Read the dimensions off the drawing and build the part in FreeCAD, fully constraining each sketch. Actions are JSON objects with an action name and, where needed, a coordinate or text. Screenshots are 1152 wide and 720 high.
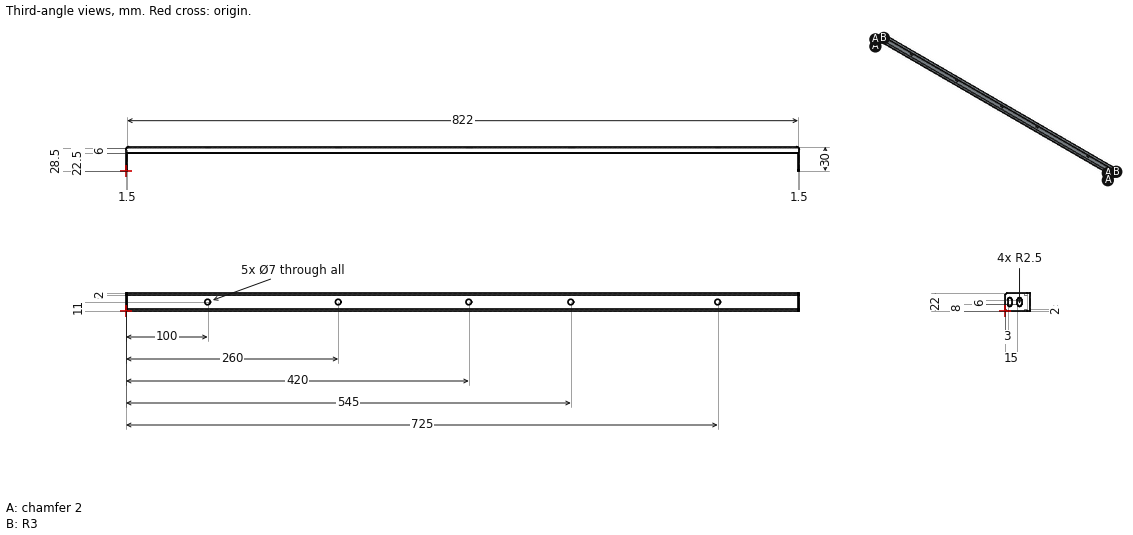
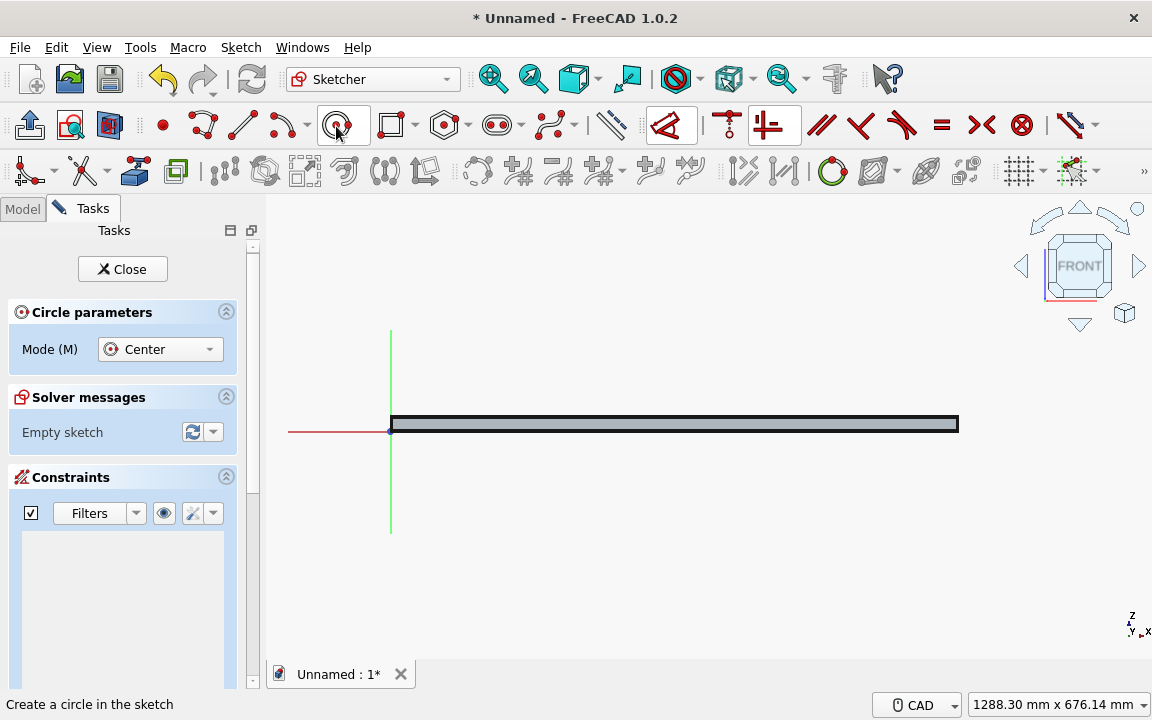
{"action": "scroll", "coordinate": [459, 424], "scroll_direction": "up", "scroll_amount": 12}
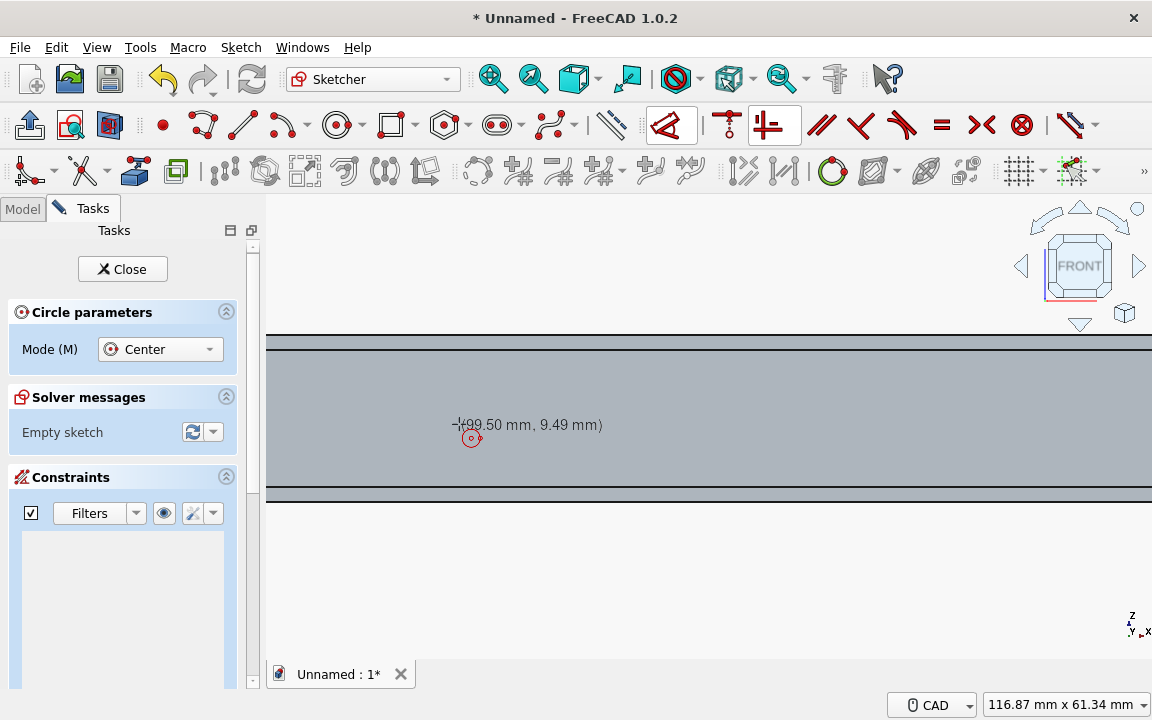
{"action": "scroll", "coordinate": [459, 424], "scroll_direction": "down", "scroll_amount": 12}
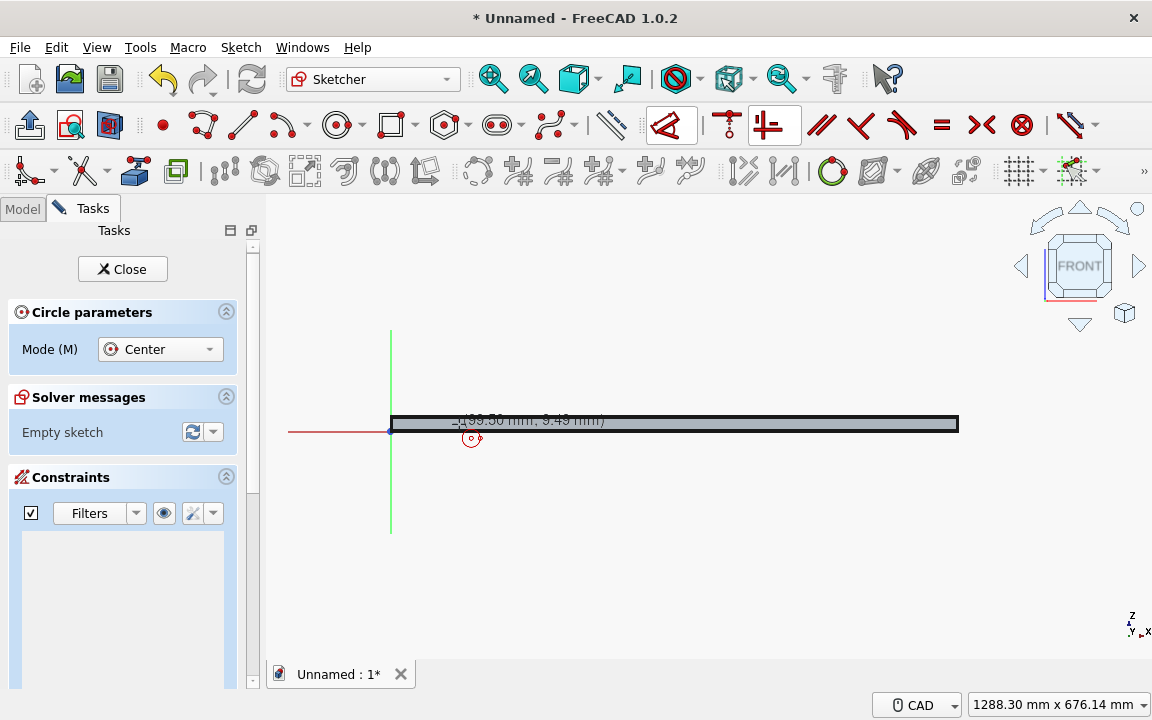
{"action": "scroll", "coordinate": [459, 424], "scroll_direction": "up", "scroll_amount": 4}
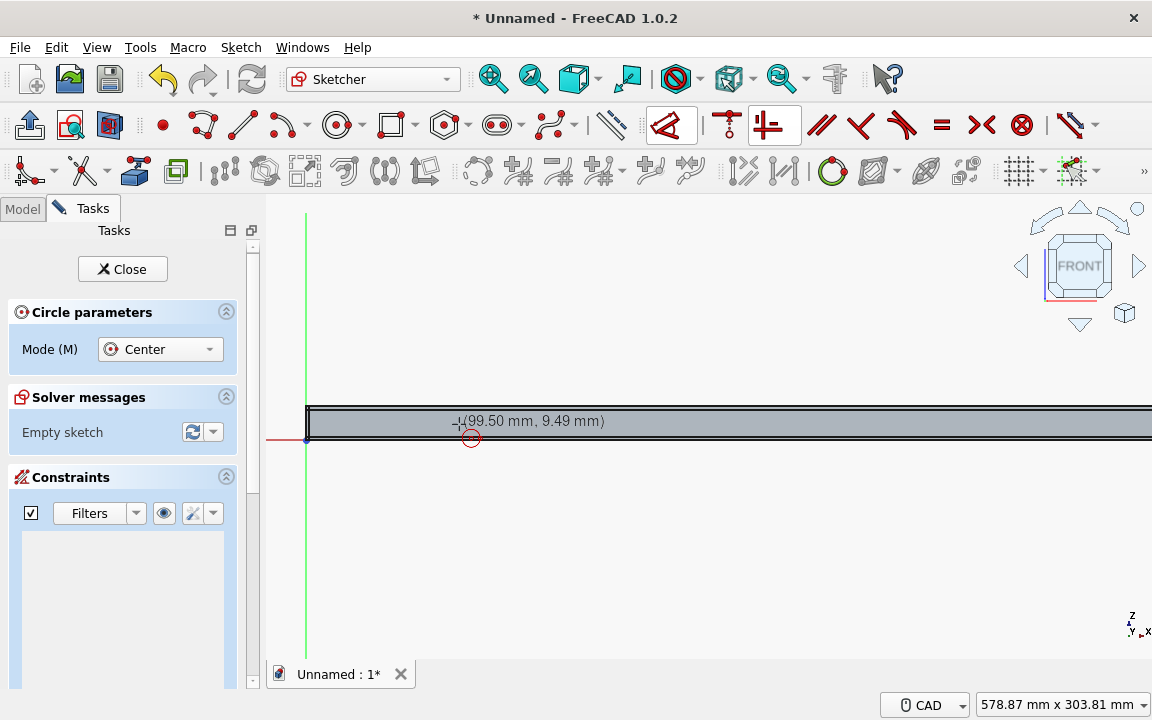
{"action": "left_click", "coordinate": [460, 423]}
{"action": "mouse_move", "coordinate": [463, 420]}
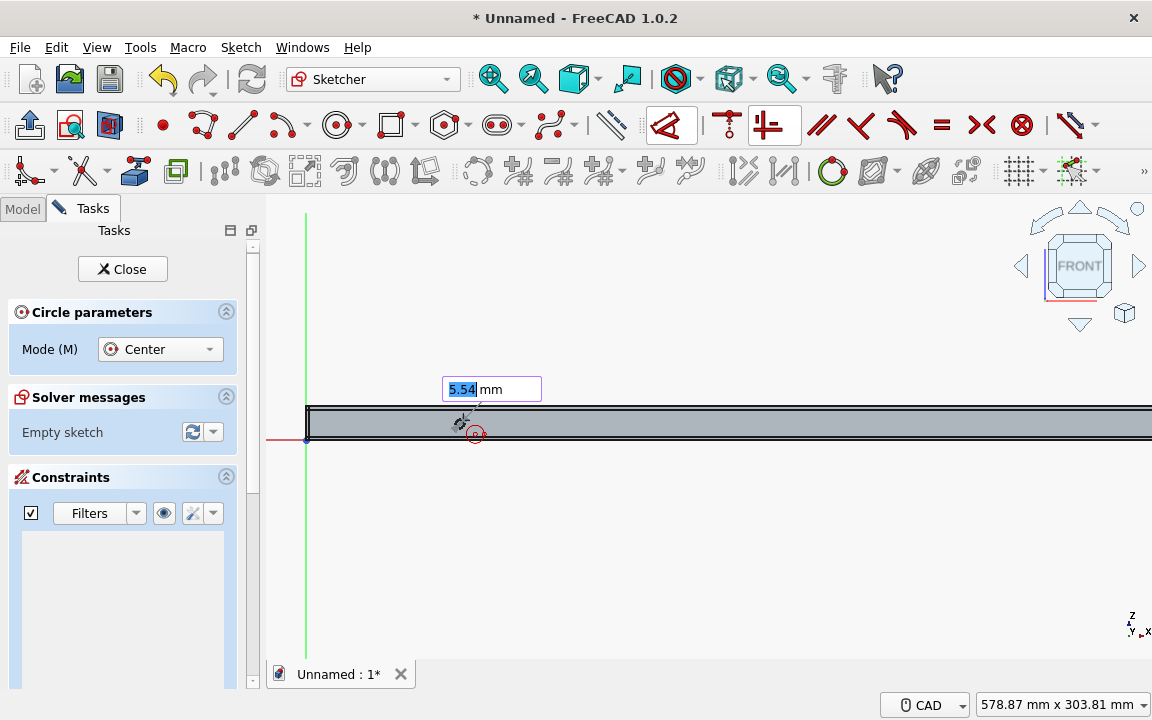
{"action": "type", "text": "7"}
{"action": "key", "text": "Return"}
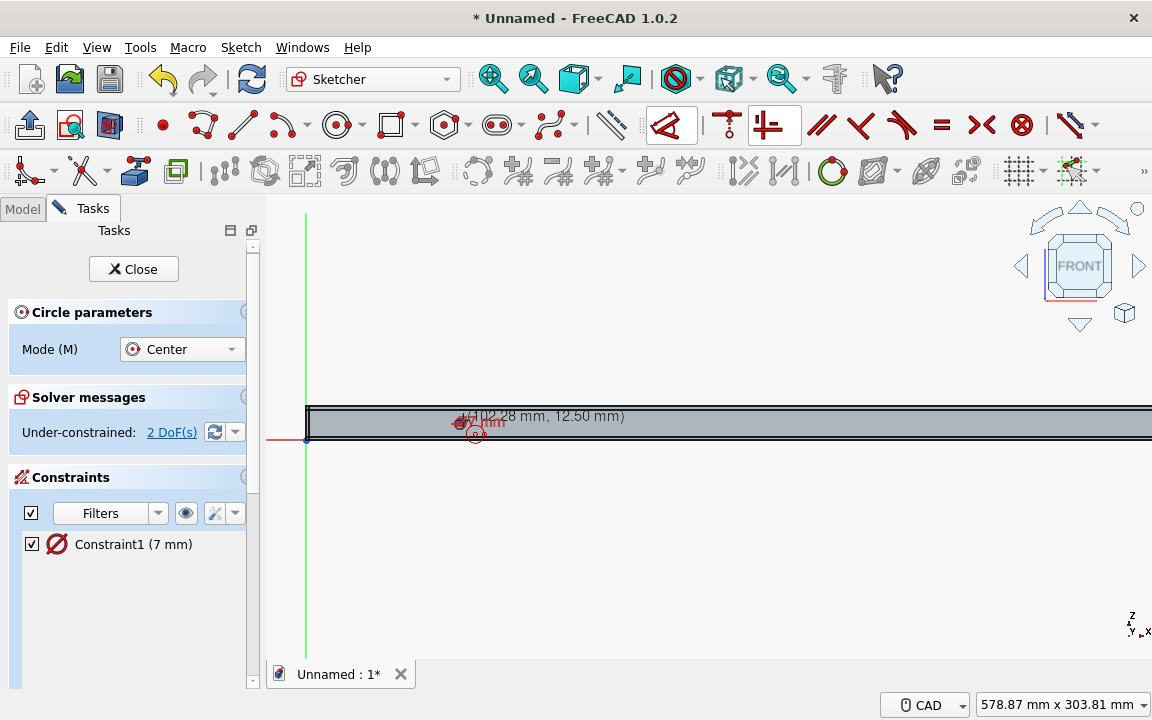
{"action": "scroll", "coordinate": [704, 423], "scroll_direction": "up", "scroll_amount": 8}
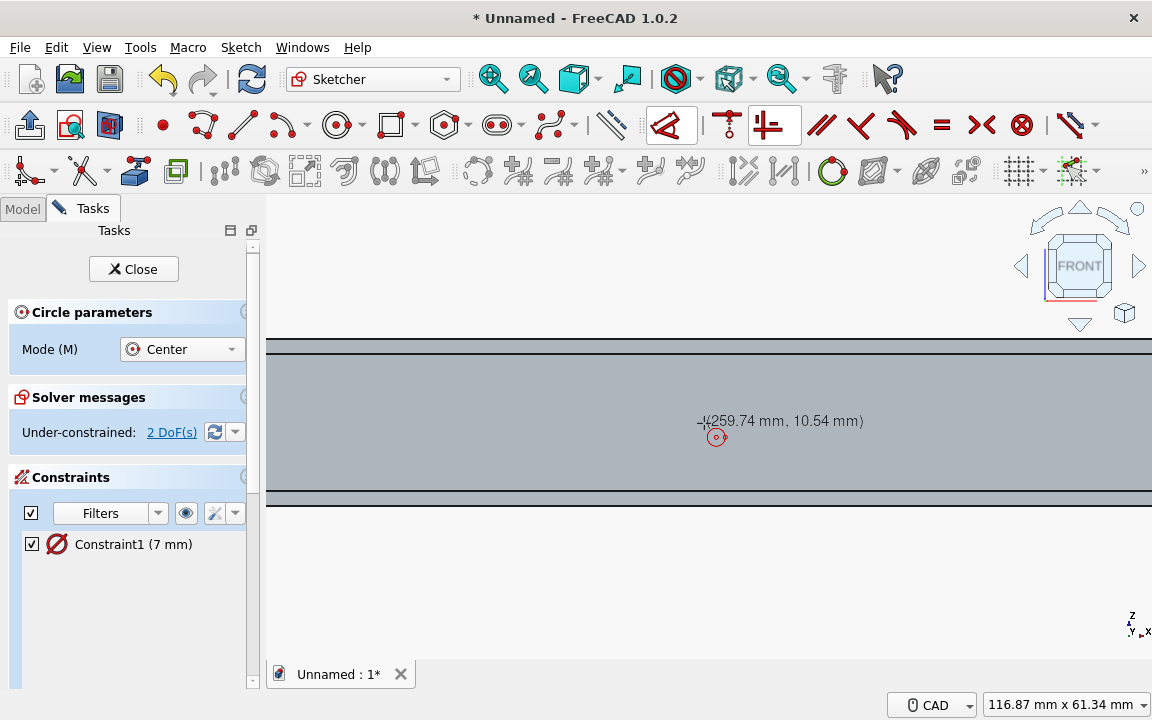
{"action": "scroll", "coordinate": [555, 424], "scroll_direction": "down", "scroll_amount": 12}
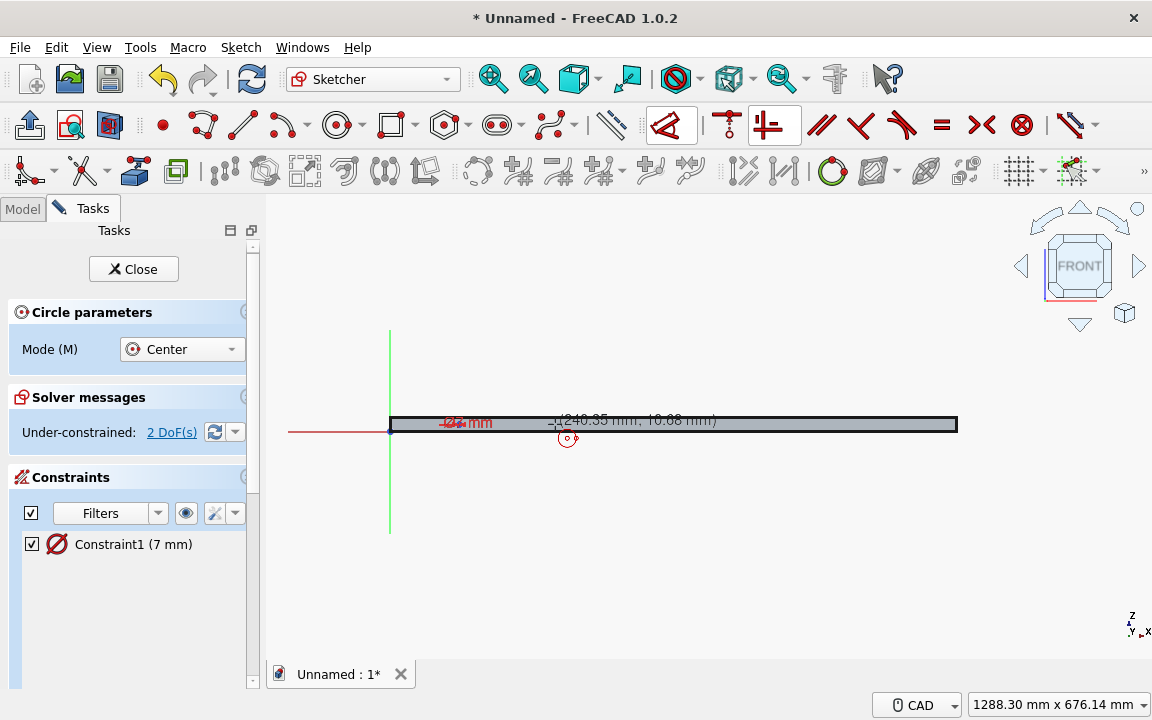
{"action": "scroll", "coordinate": [569, 424], "scroll_direction": "up", "scroll_amount": 4}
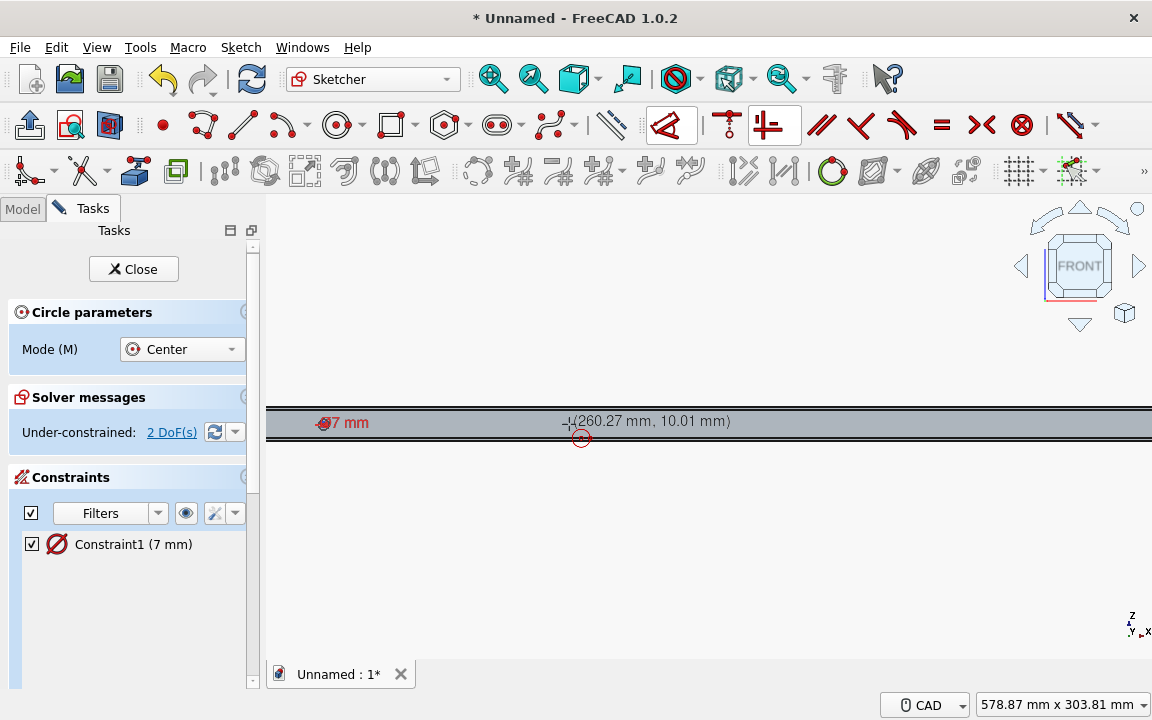
{"action": "left_click", "coordinate": [568, 424]}
{"action": "mouse_move", "coordinate": [572, 420]}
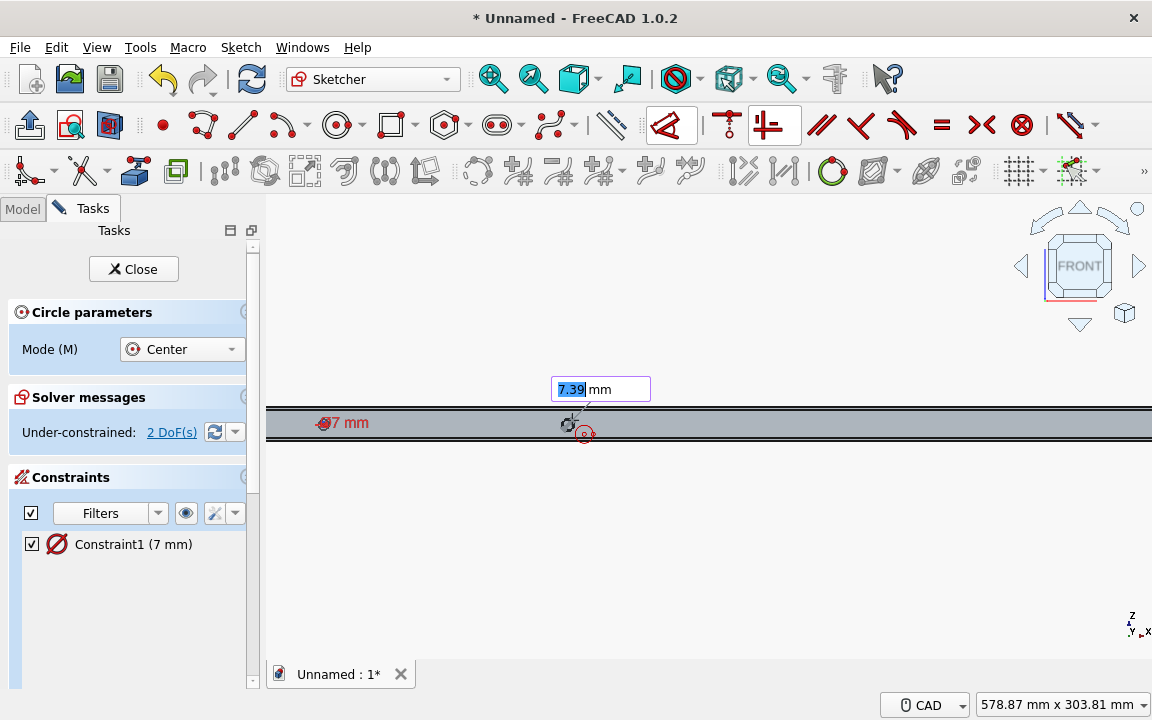
{"action": "type", "text": "7"}
{"action": "key", "text": "Return"}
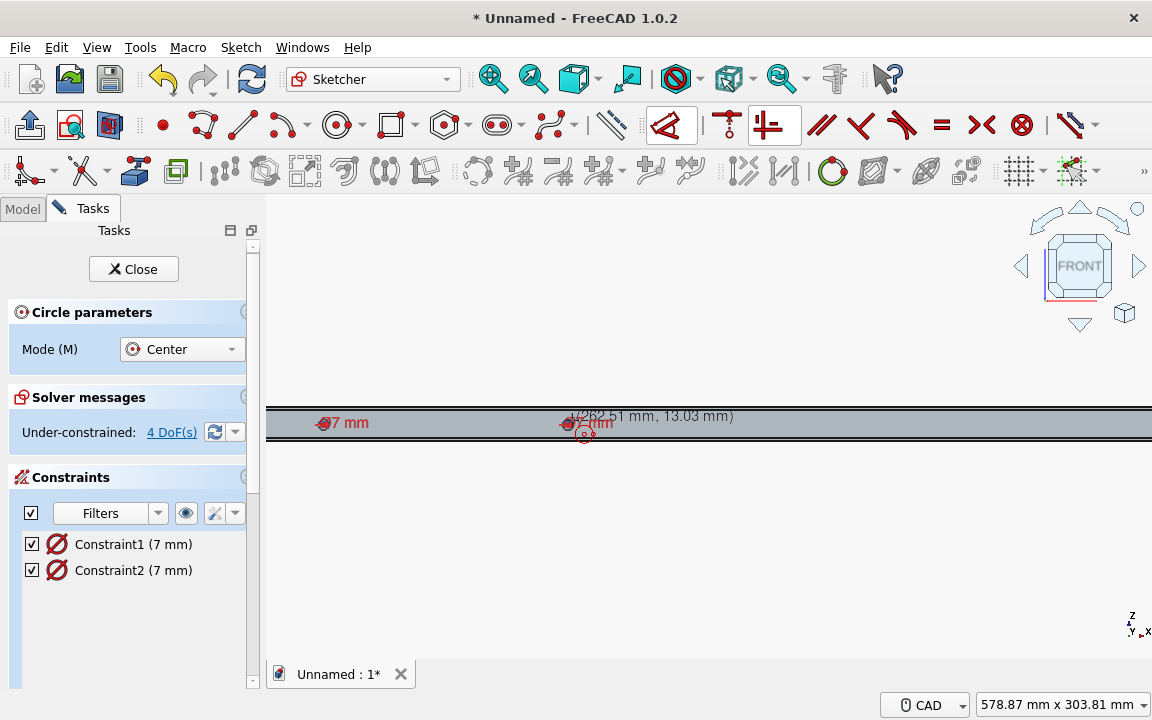
{"action": "scroll", "coordinate": [813, 424], "scroll_direction": "up", "scroll_amount": 8}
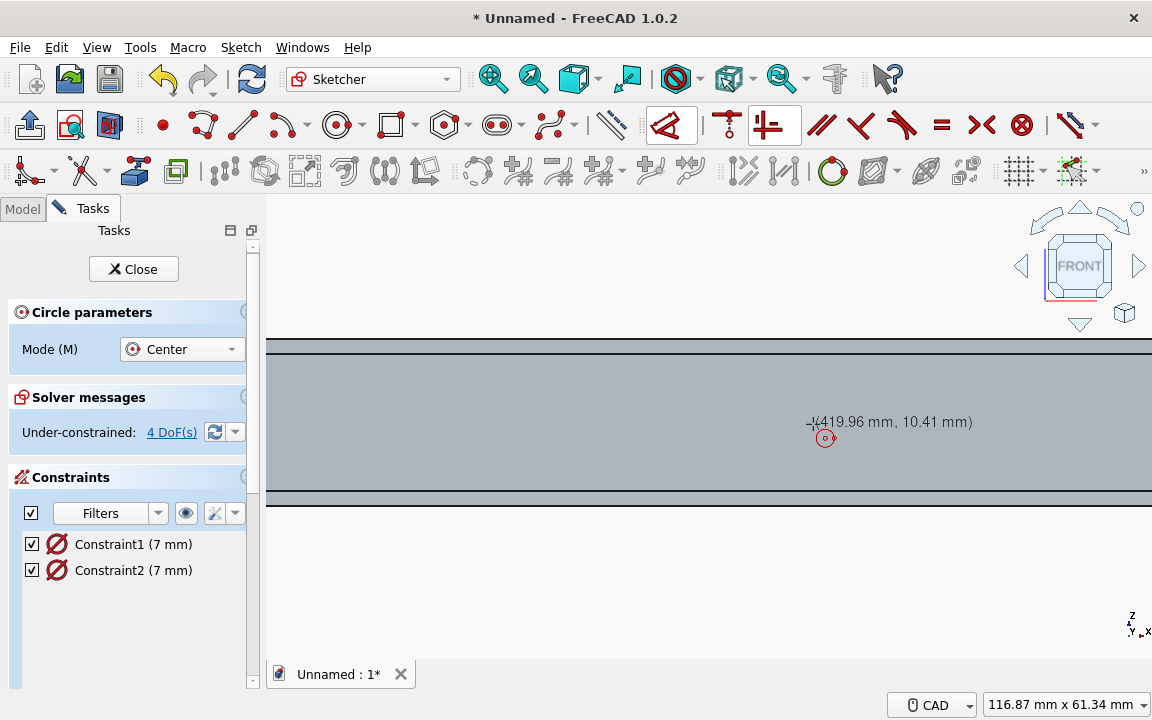
{"action": "scroll", "coordinate": [666, 424], "scroll_direction": "down", "scroll_amount": 12}